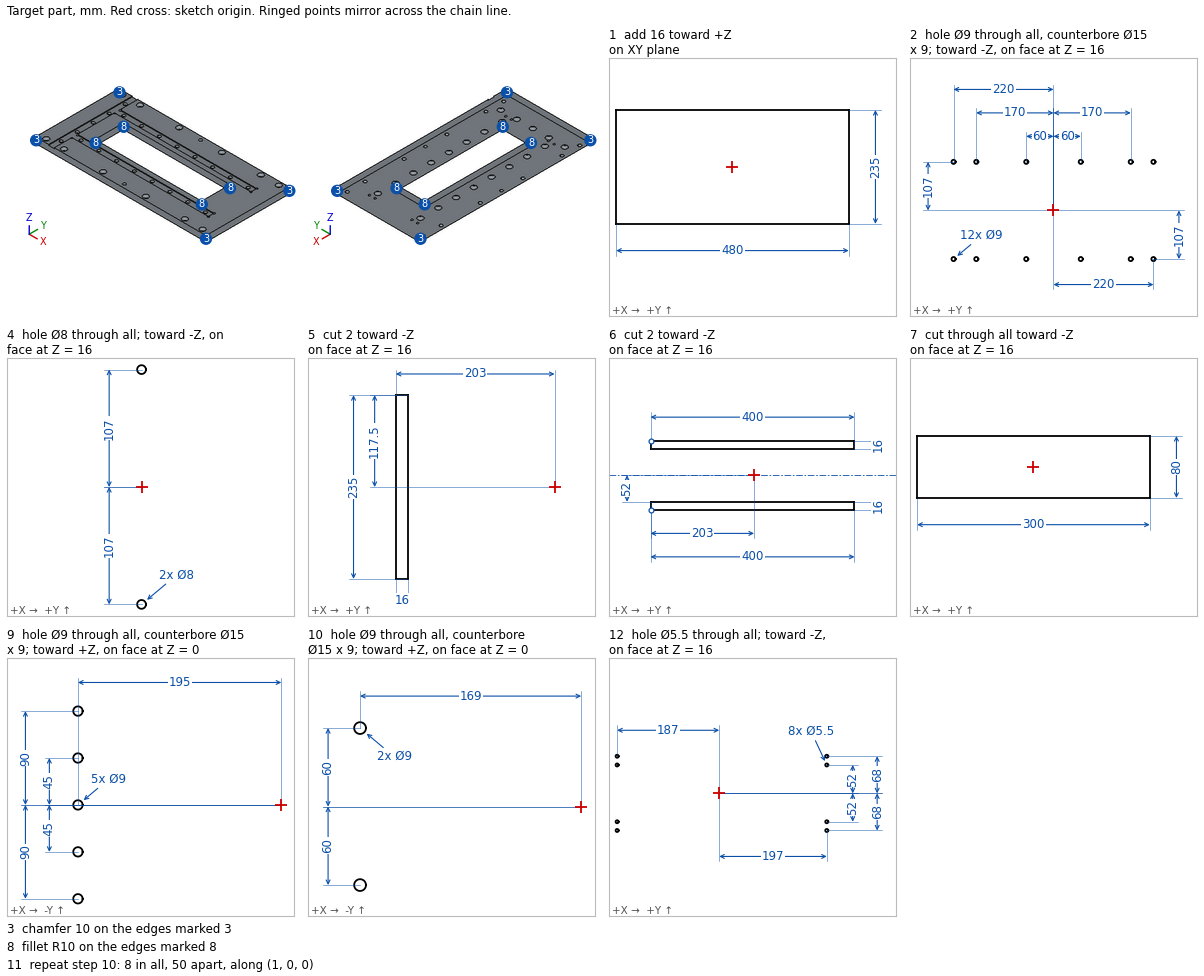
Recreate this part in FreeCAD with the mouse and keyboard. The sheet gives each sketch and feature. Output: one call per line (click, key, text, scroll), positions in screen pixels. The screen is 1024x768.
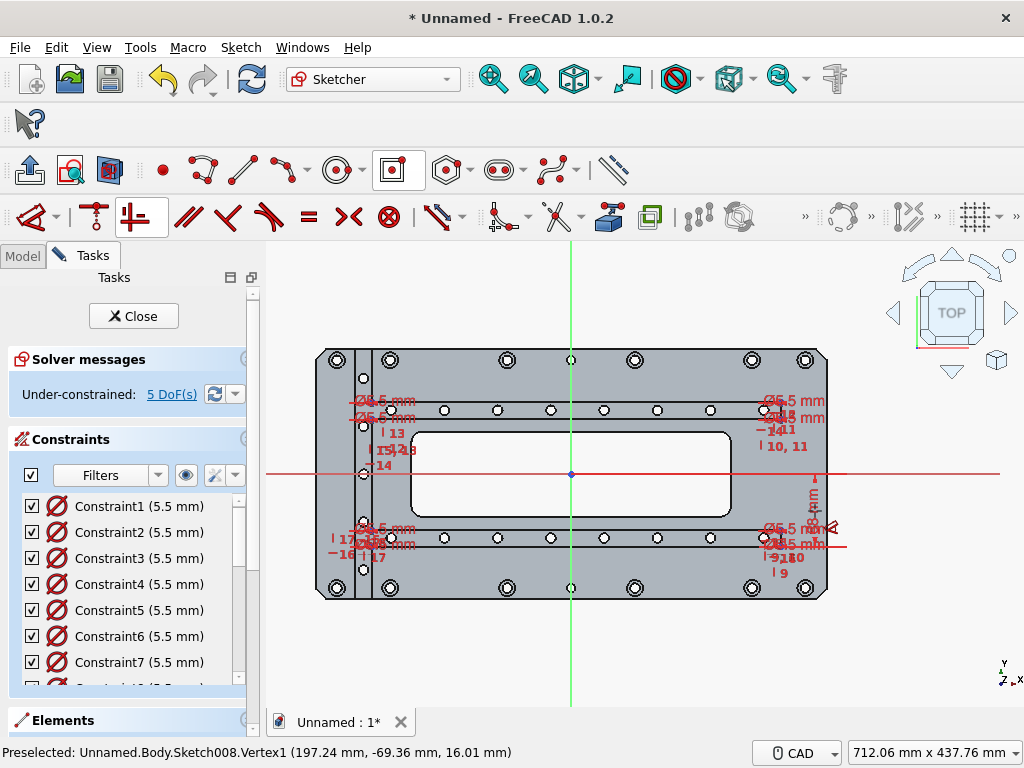
click(781, 531)
click(815, 490)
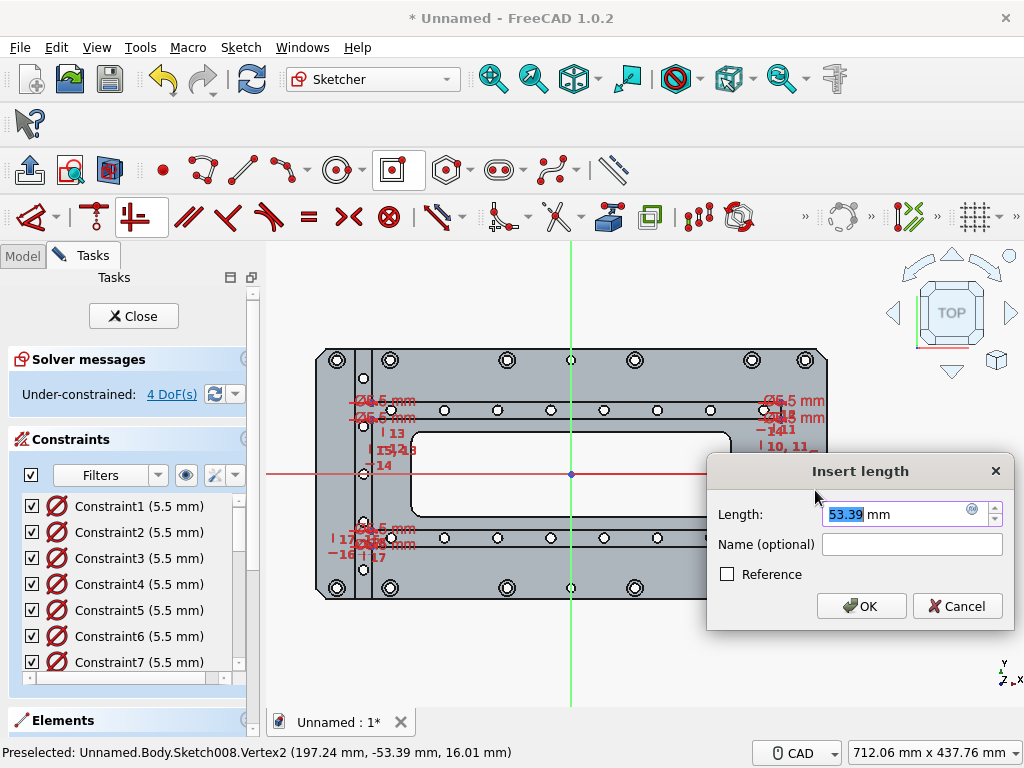
text(52)
key(Return)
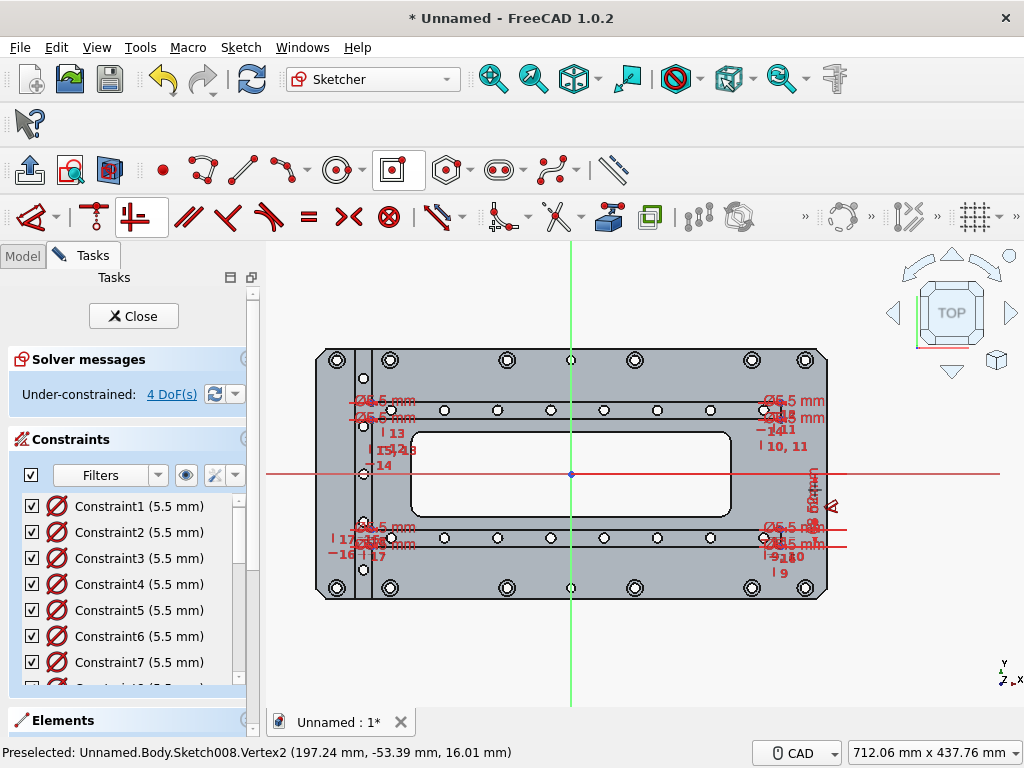
click(781, 420)
click(815, 447)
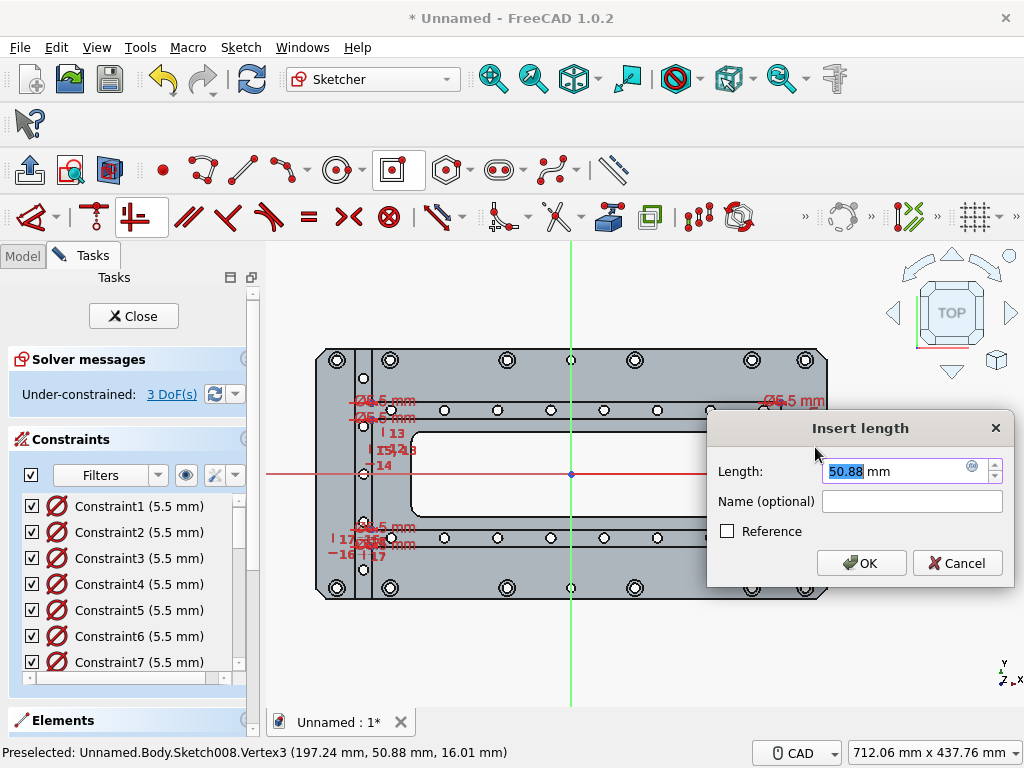
text(52)
key(Return)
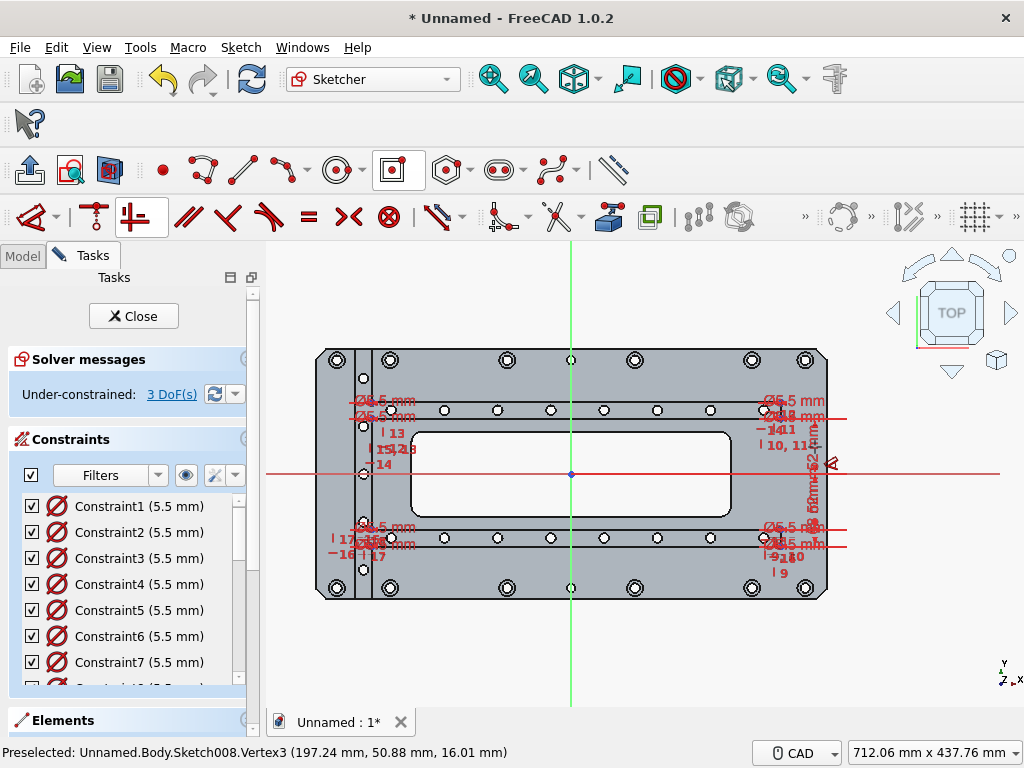
click(781, 403)
click(815, 422)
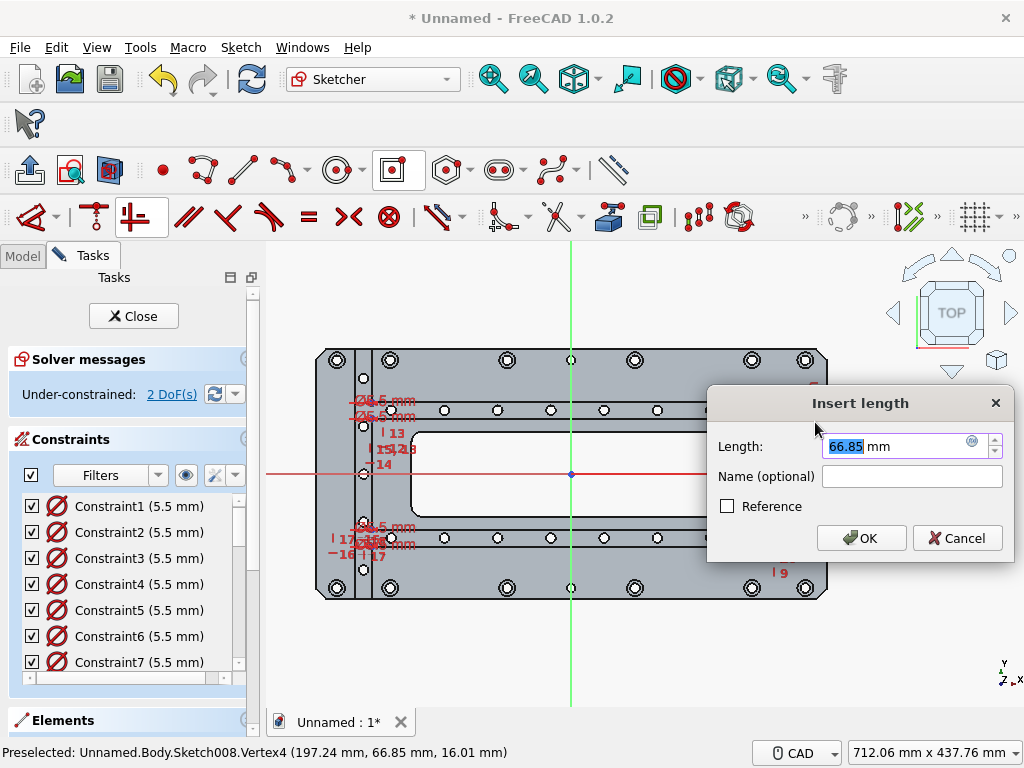
text(68)
key(Return)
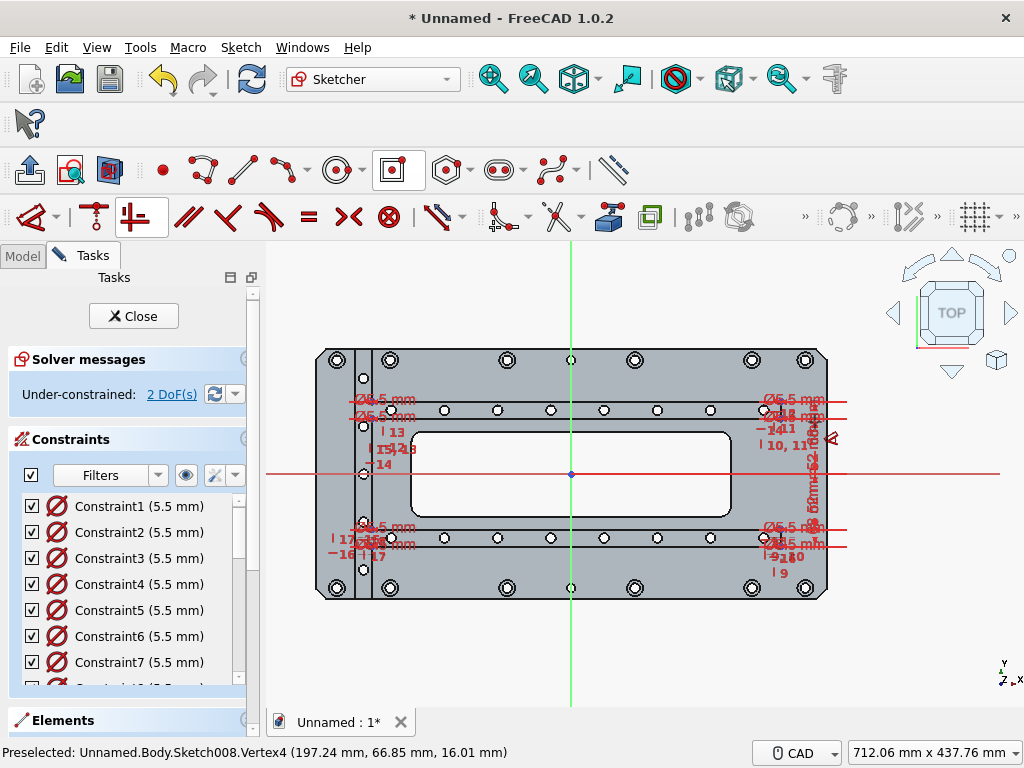
click(781, 547)
click(676, 581)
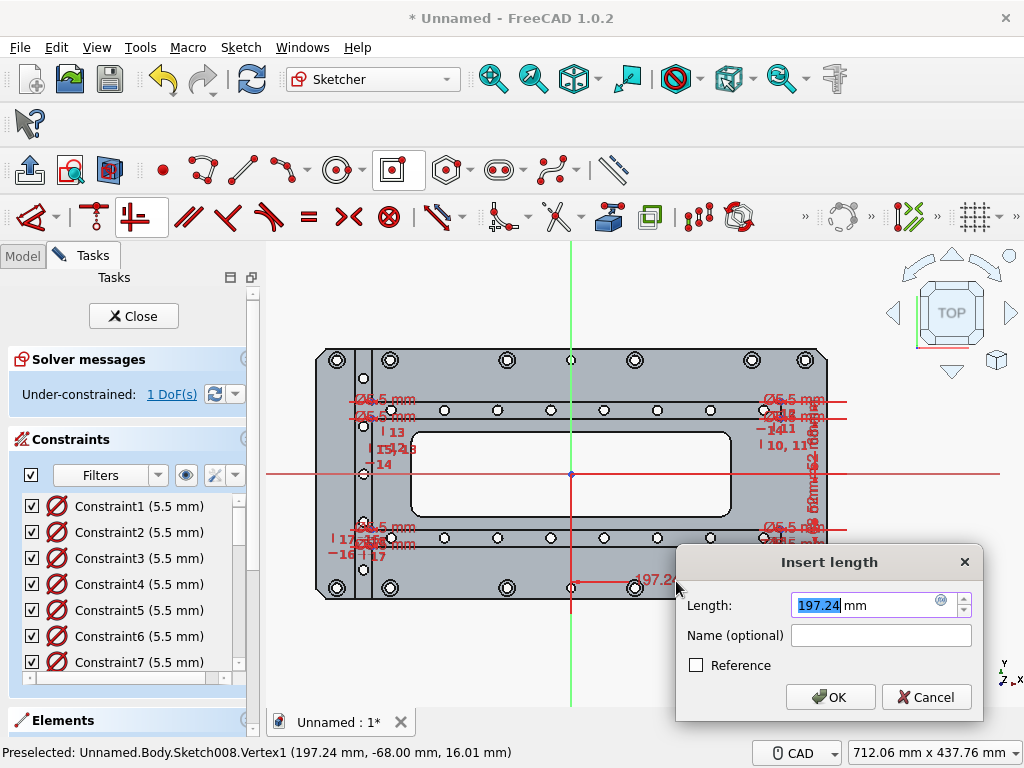
text(197)
key(Return)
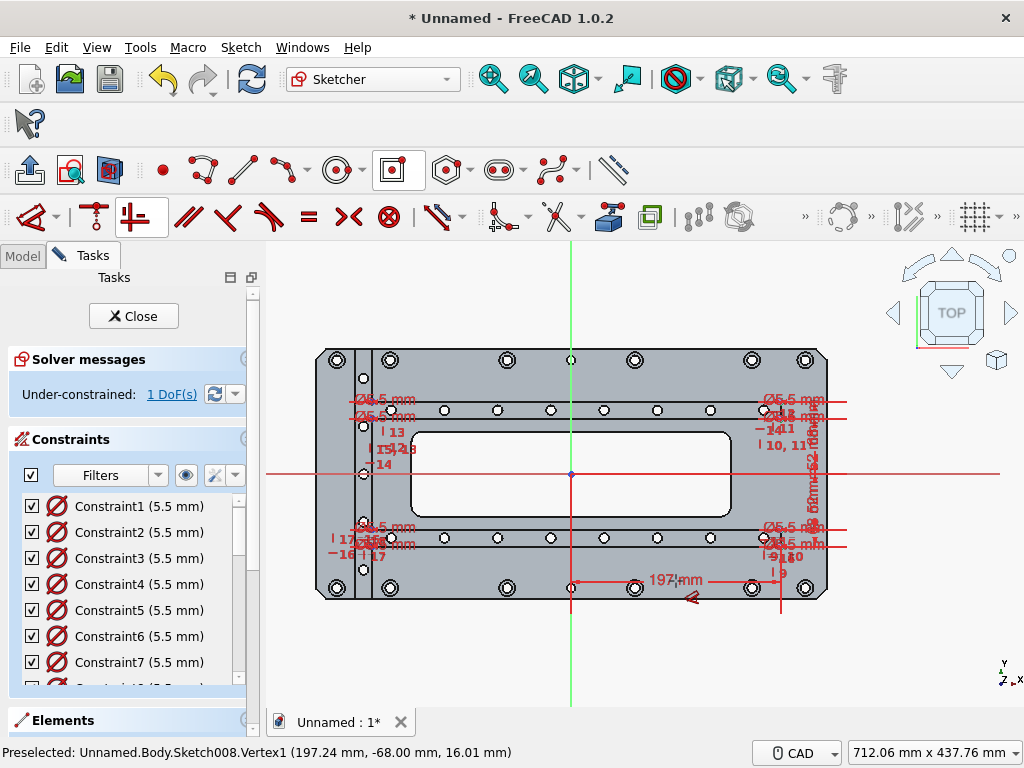
click(372, 402)
click(472, 368)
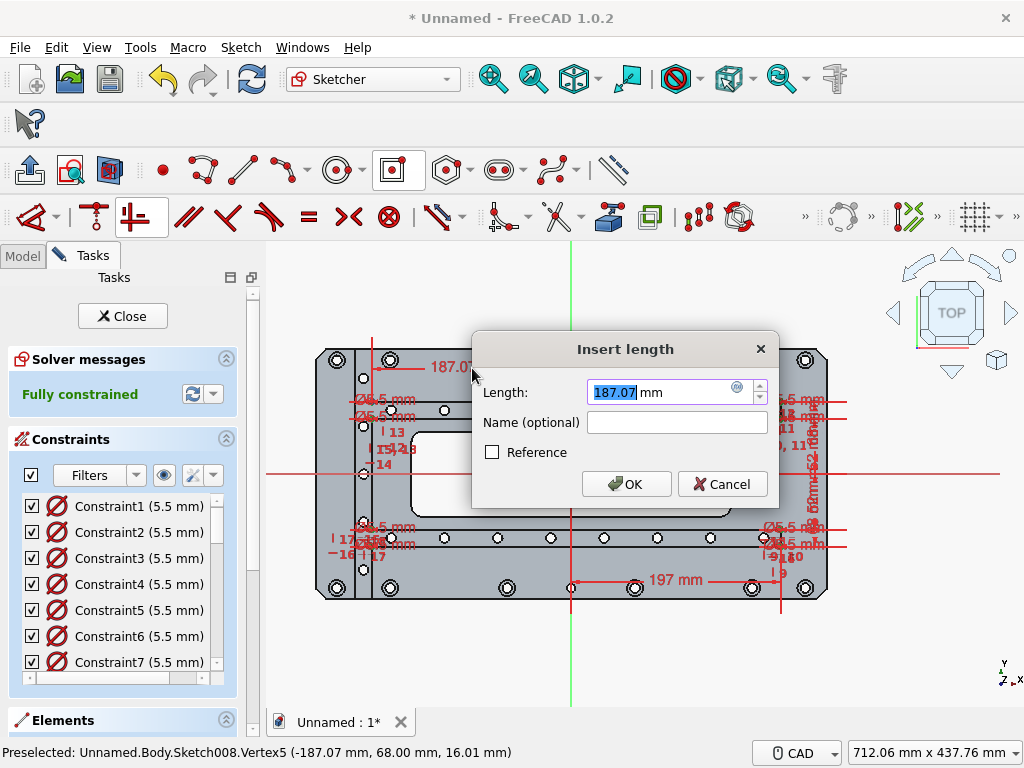
text(187)
key(Return)
key(Escape)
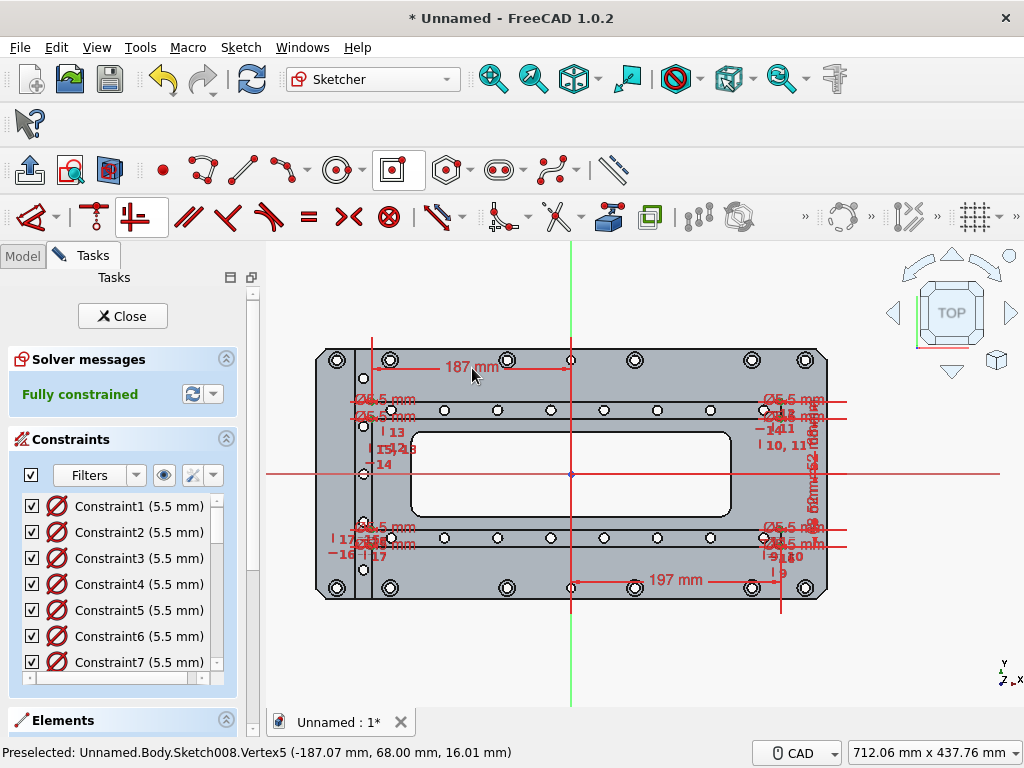
click(123, 316)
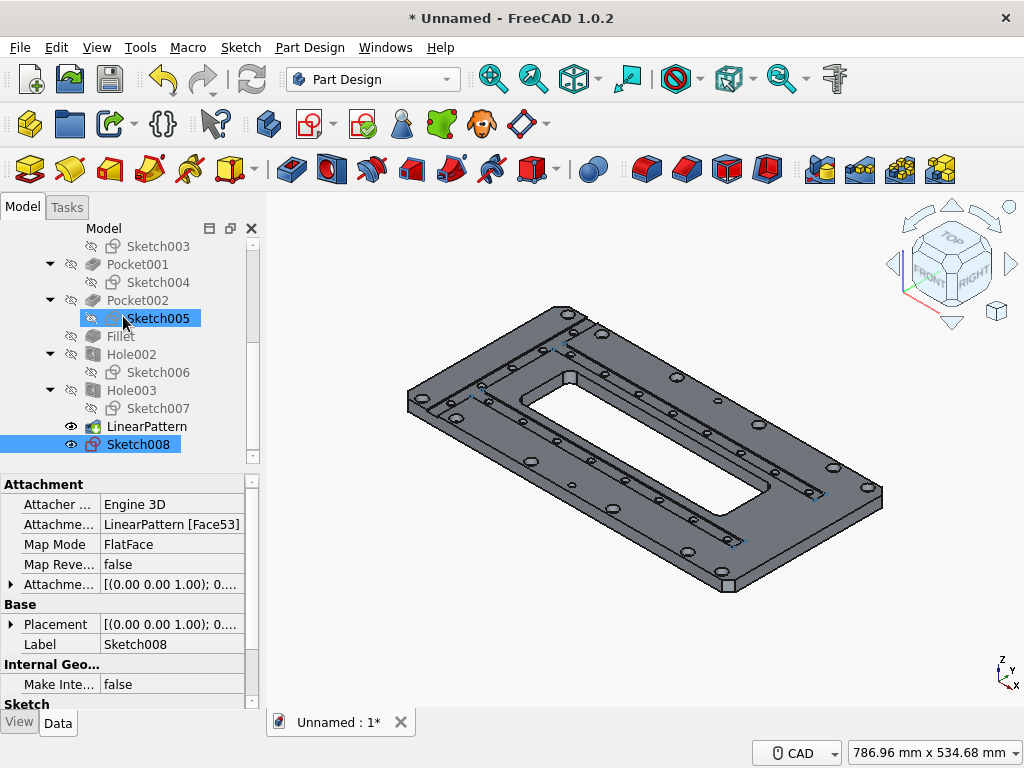
click(332, 170)